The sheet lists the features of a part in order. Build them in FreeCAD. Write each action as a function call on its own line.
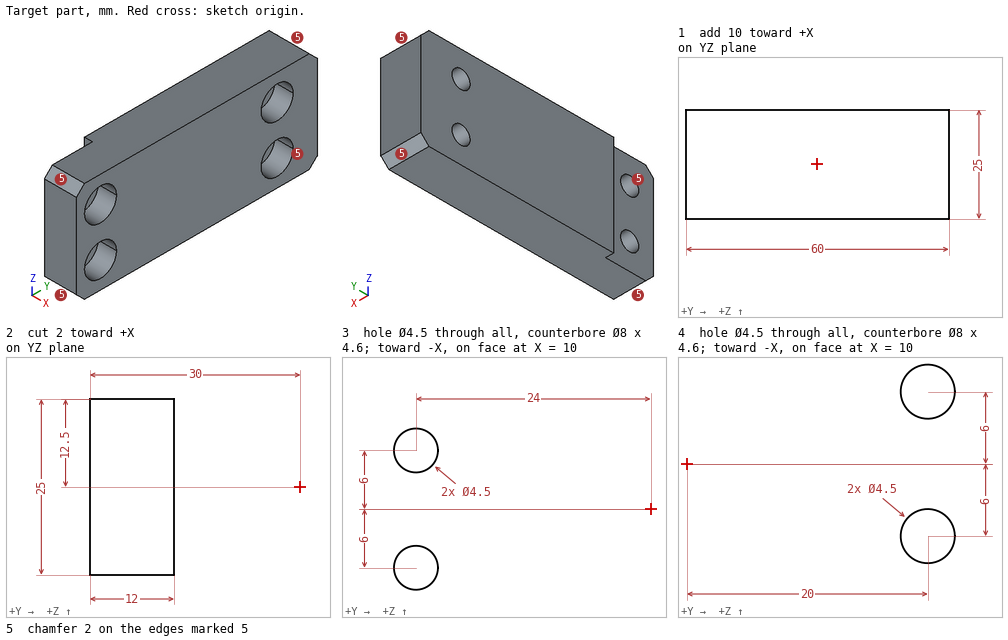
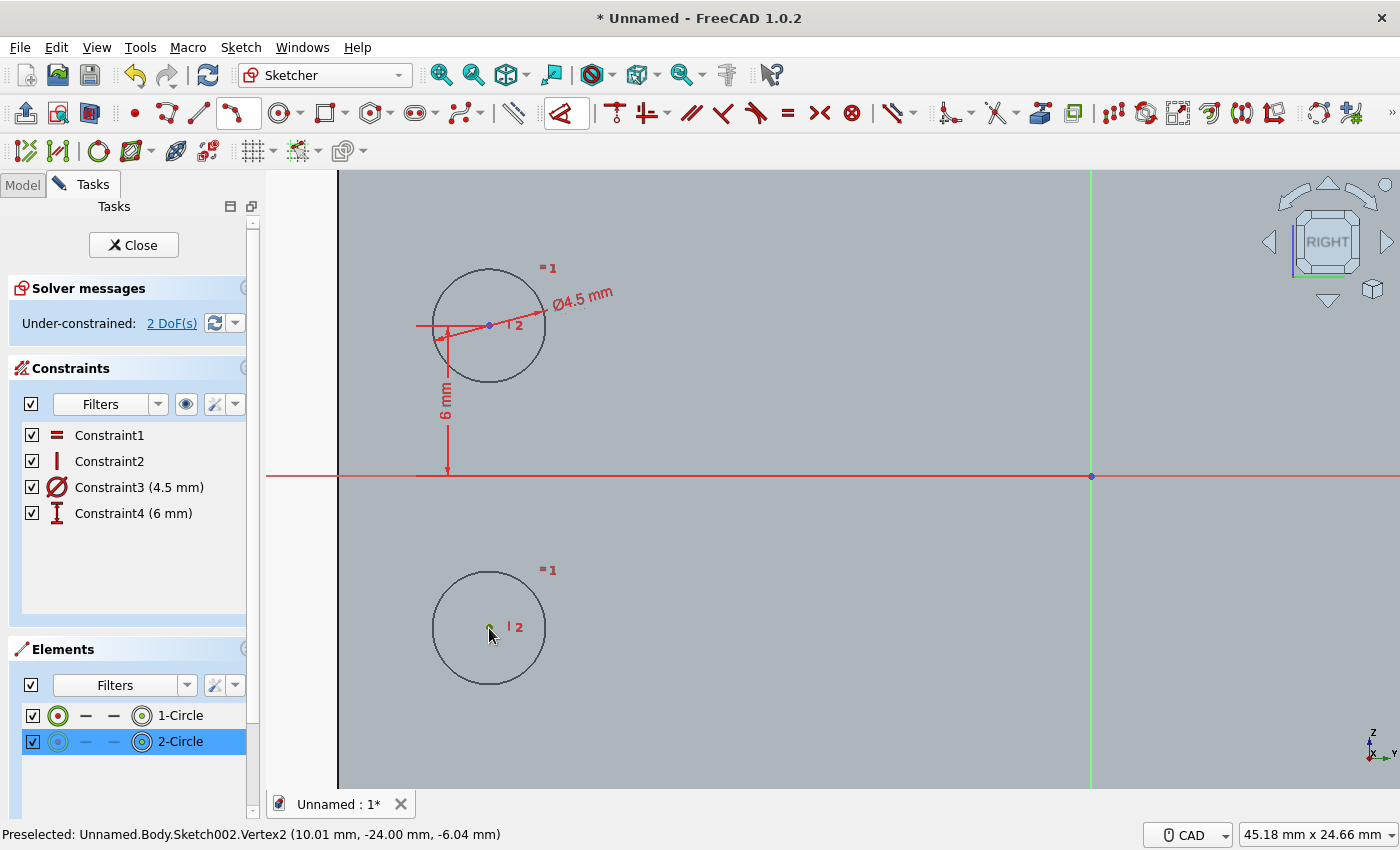
click(584, 114)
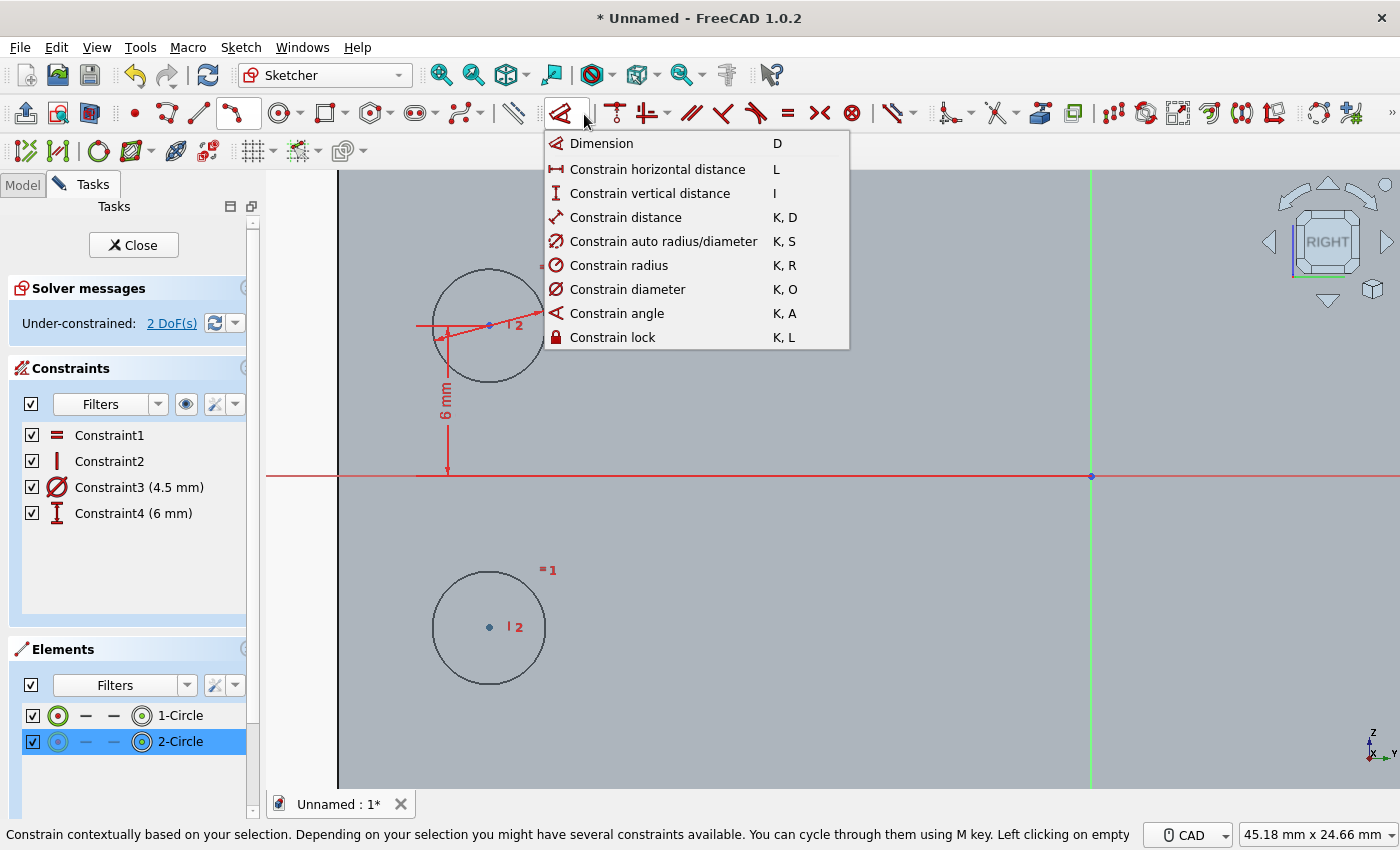
click(697, 193)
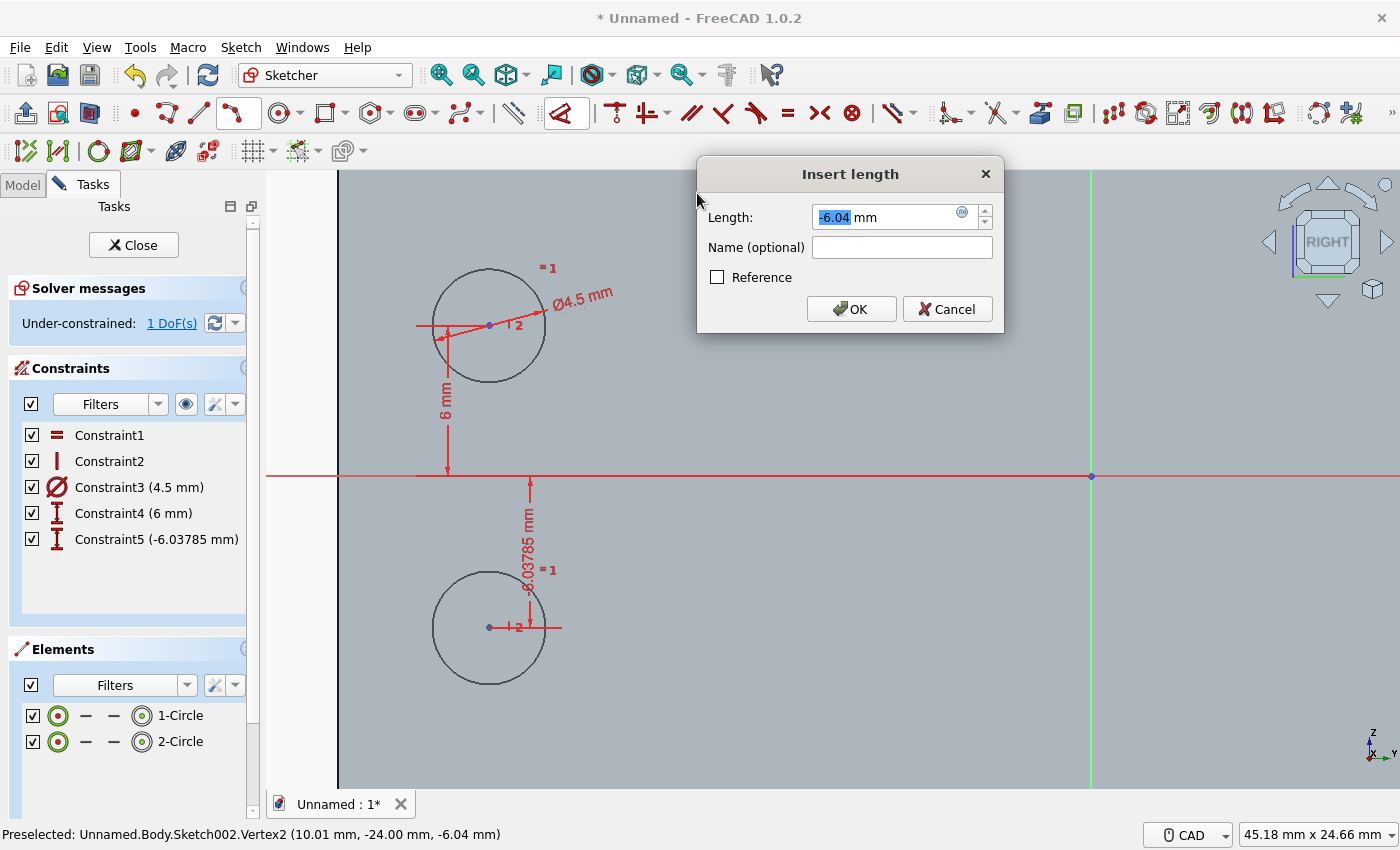
text(-6)
key(Return)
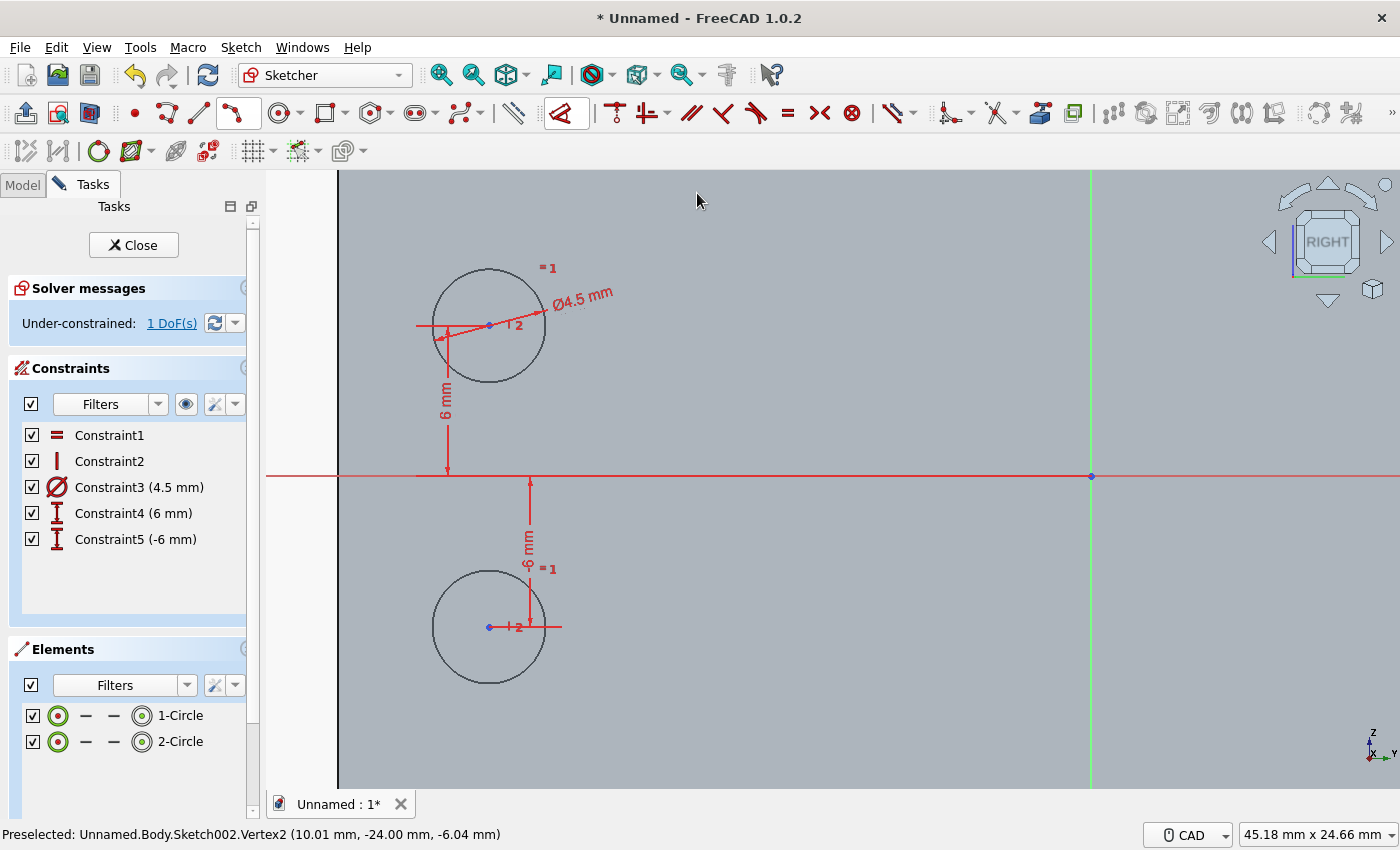
click(489, 326)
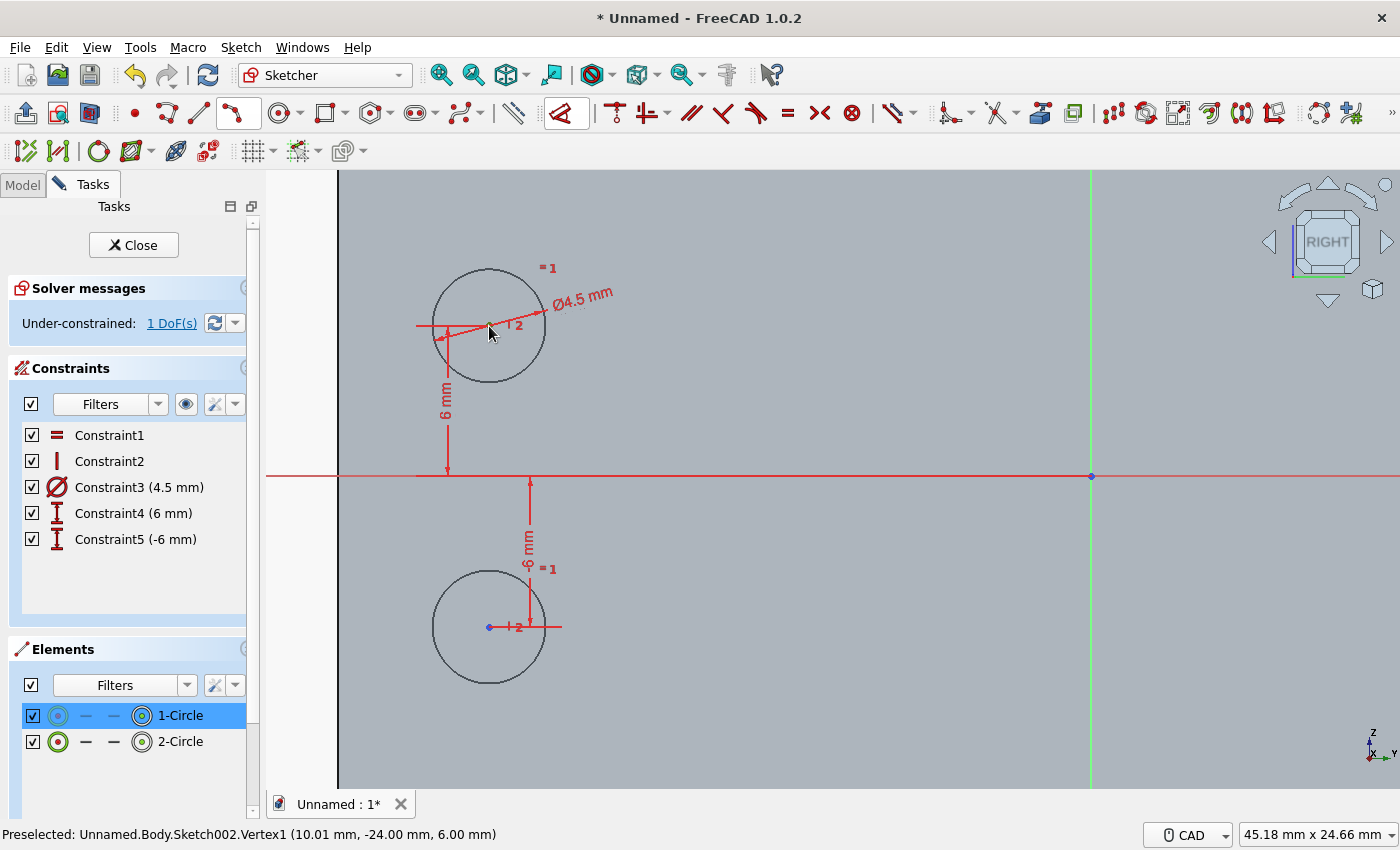
click(584, 114)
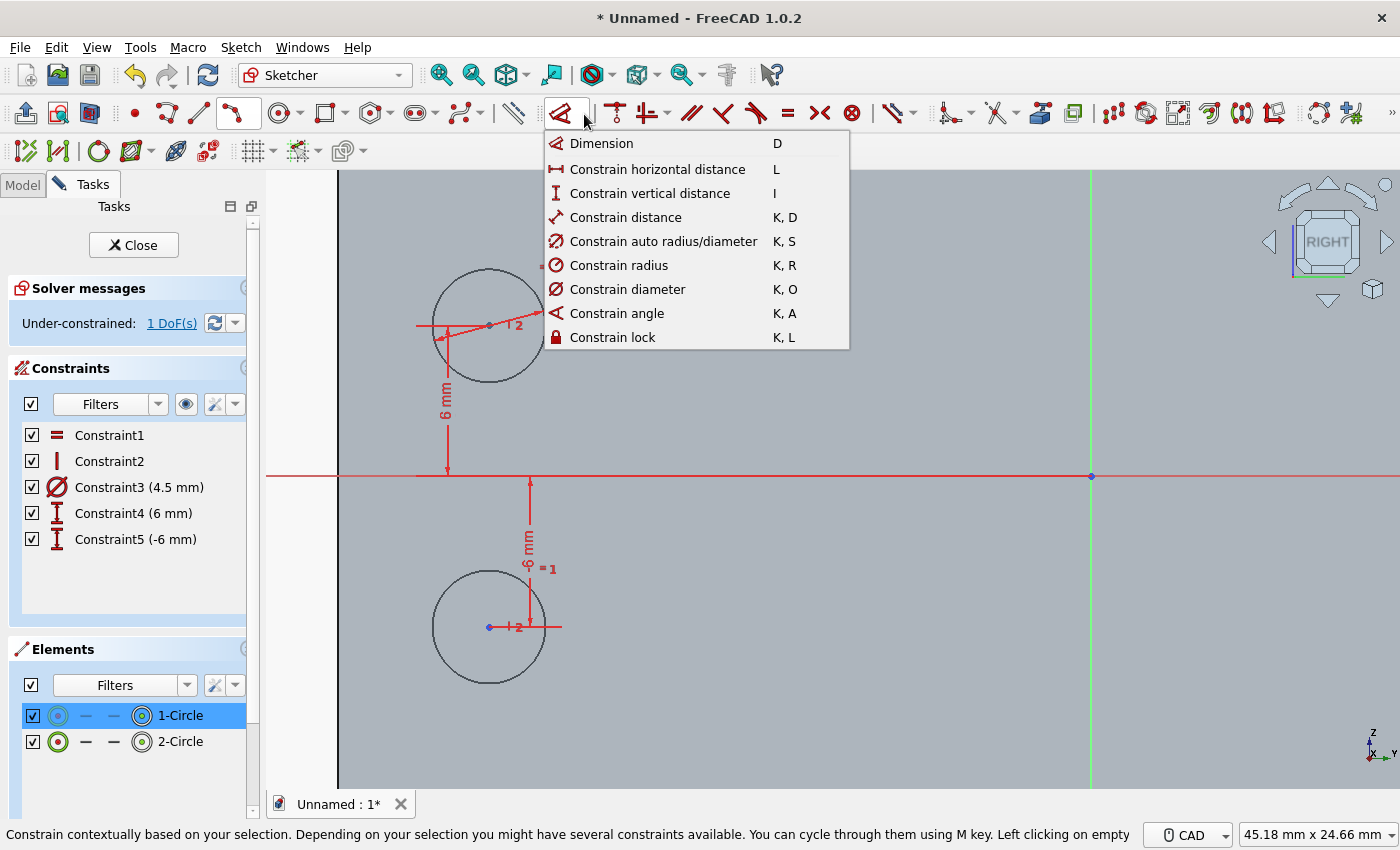
click(697, 169)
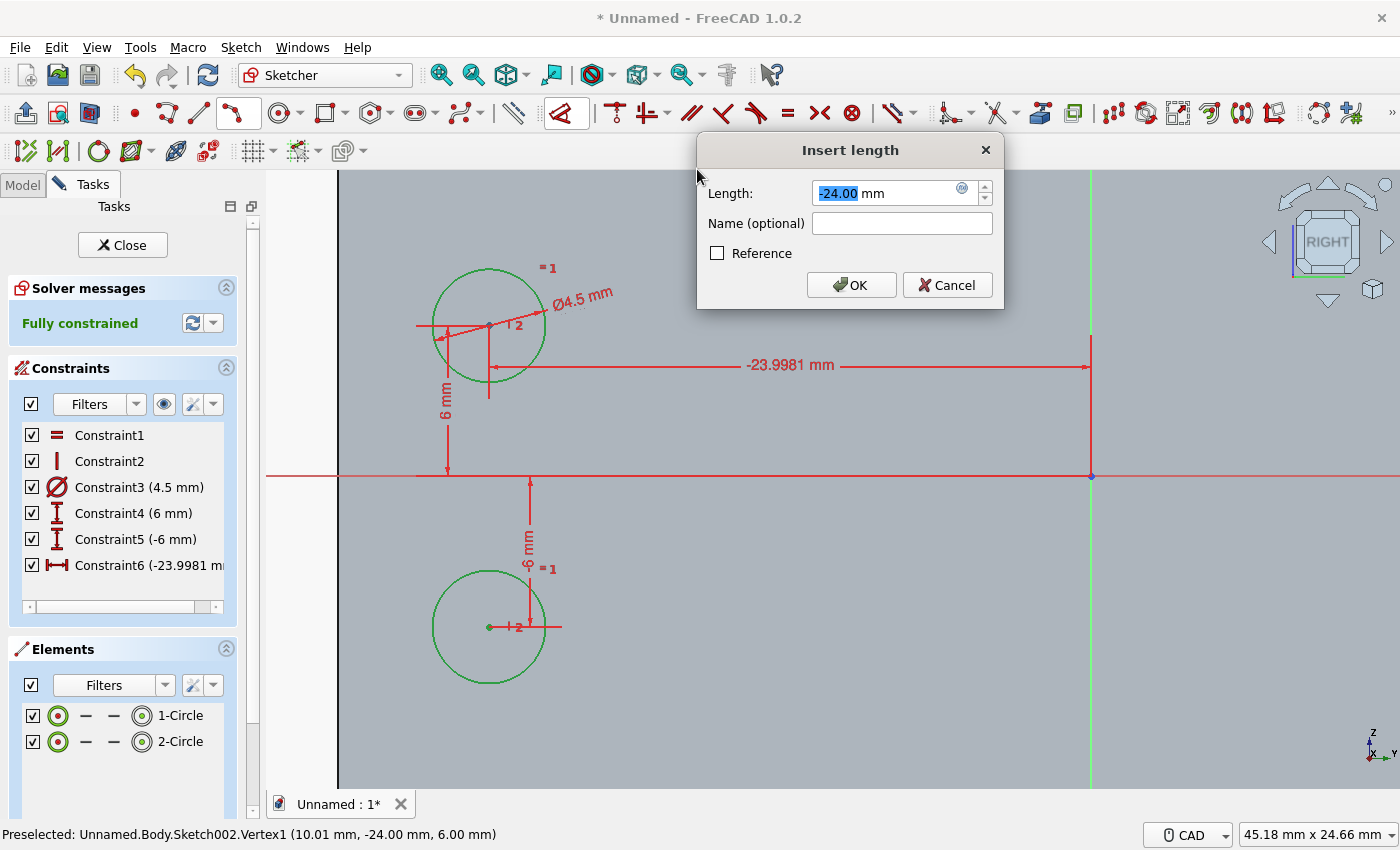
text(-24)
key(Return)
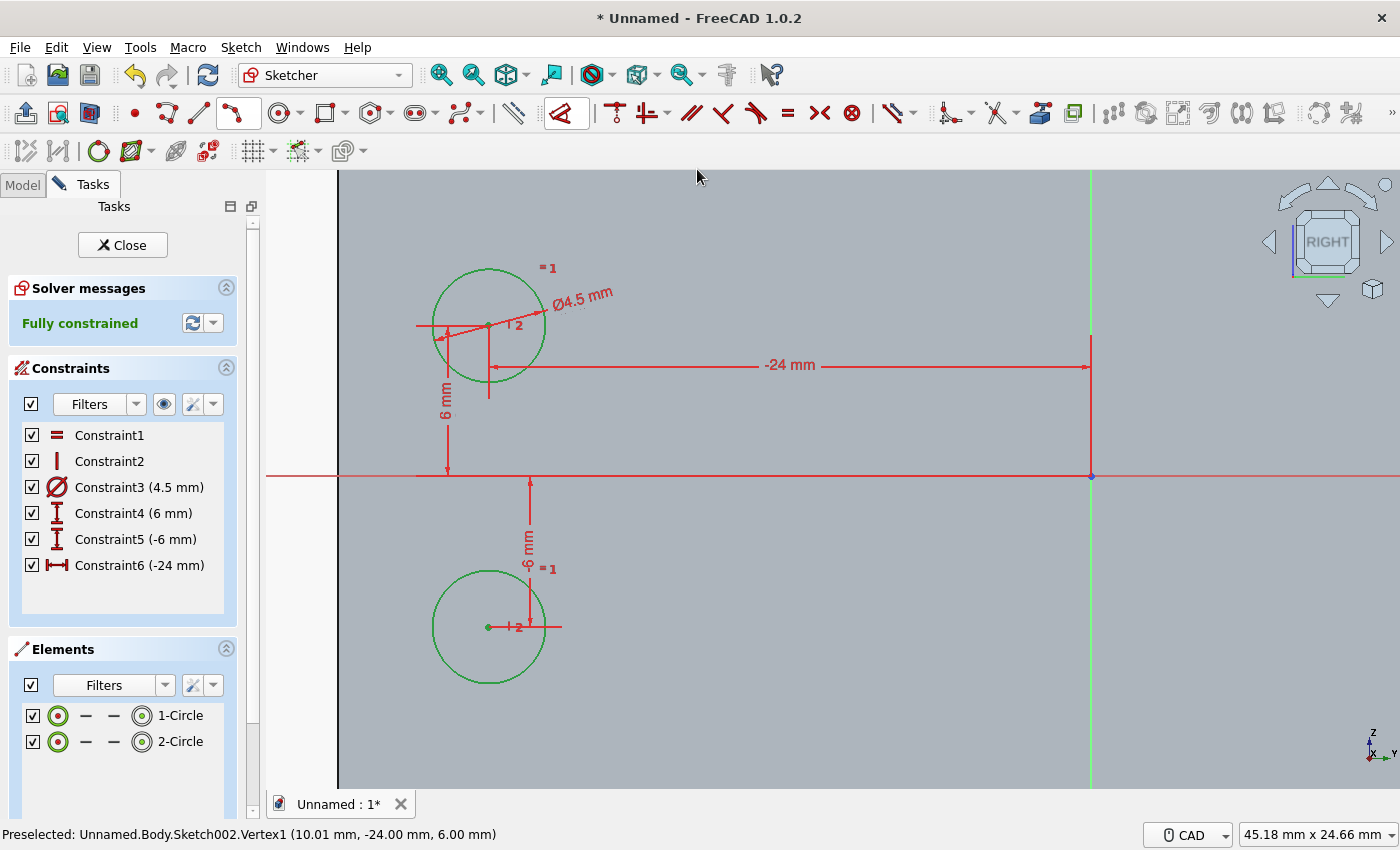
click(123, 245)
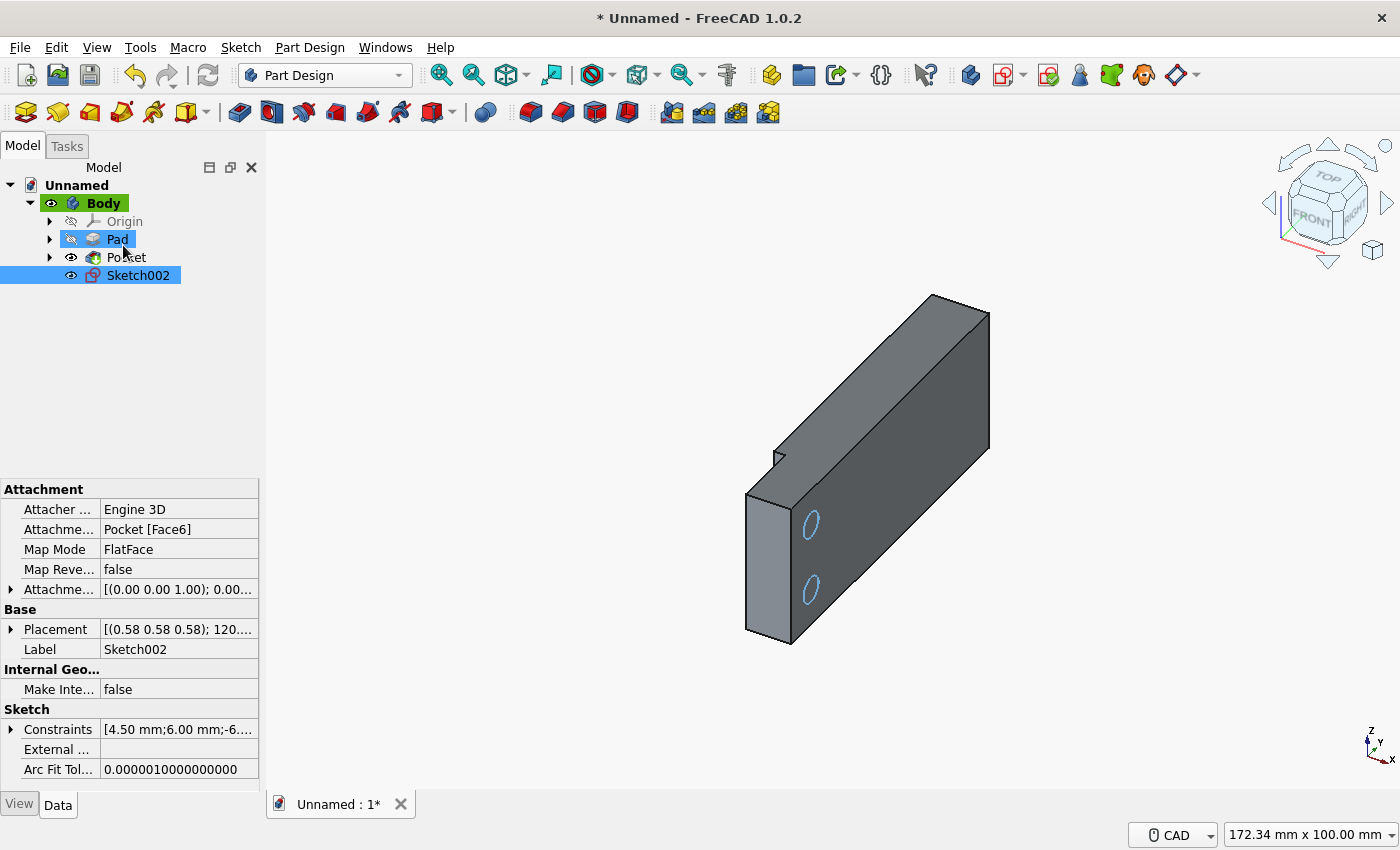
click(272, 112)